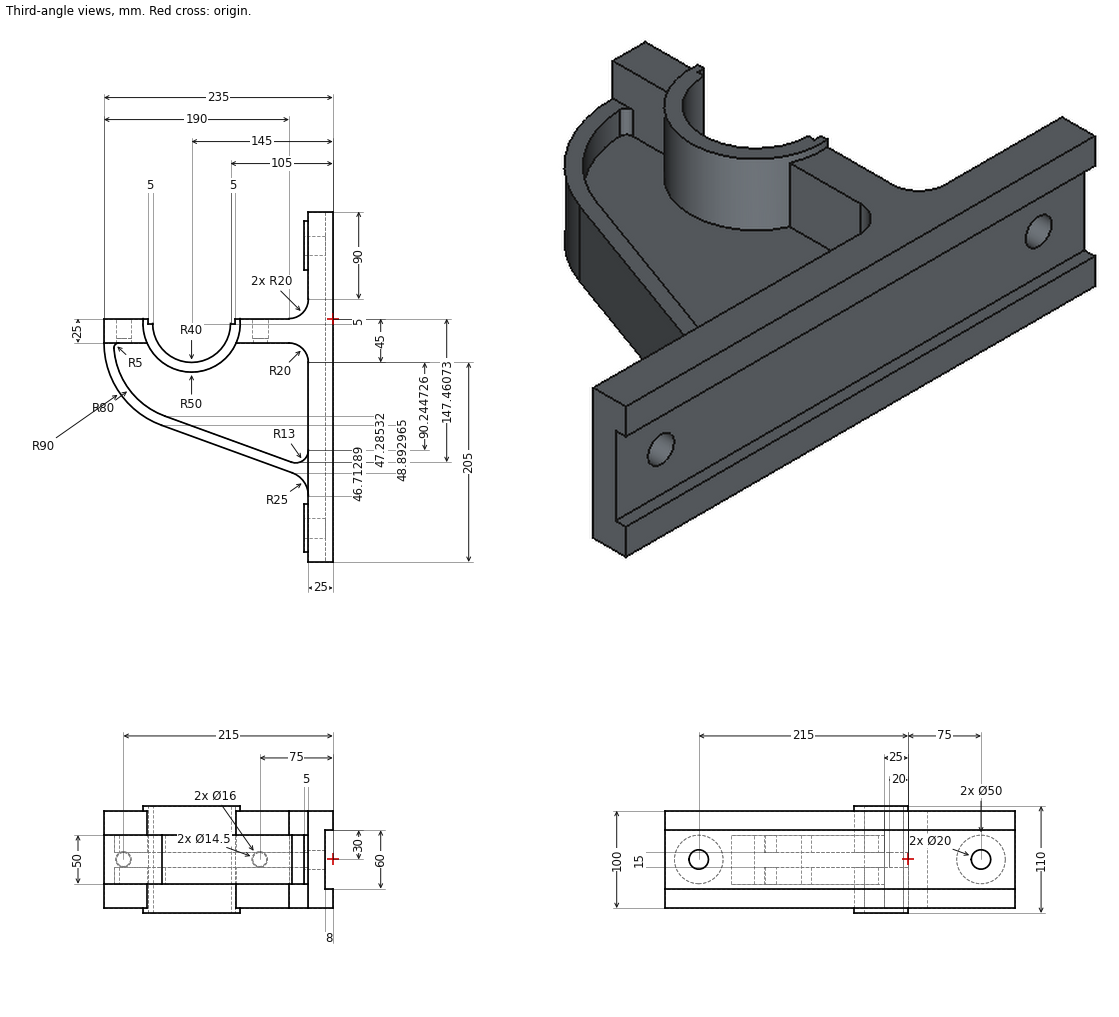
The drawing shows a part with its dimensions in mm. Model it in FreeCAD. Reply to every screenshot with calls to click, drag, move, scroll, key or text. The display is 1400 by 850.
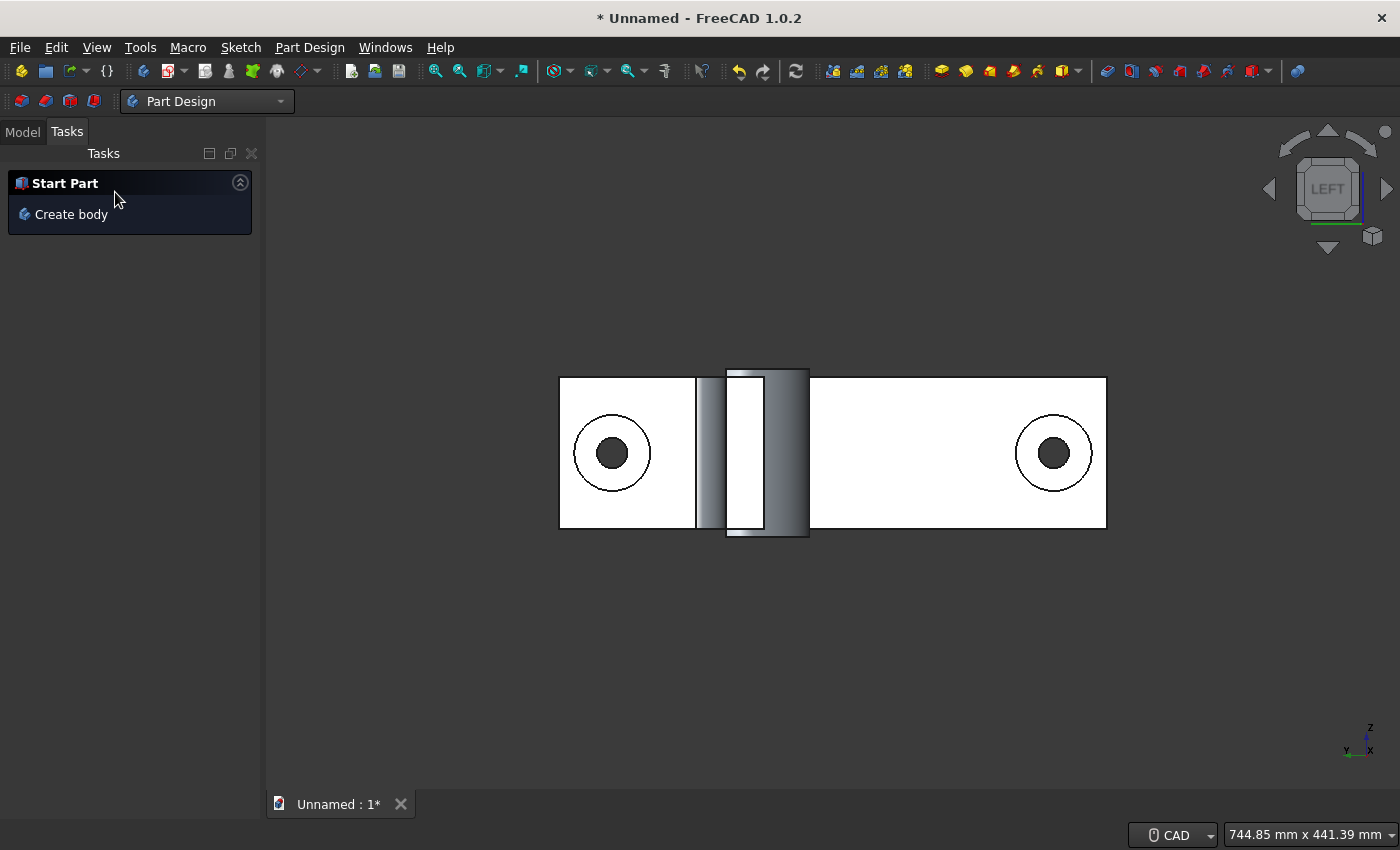
click(168, 72)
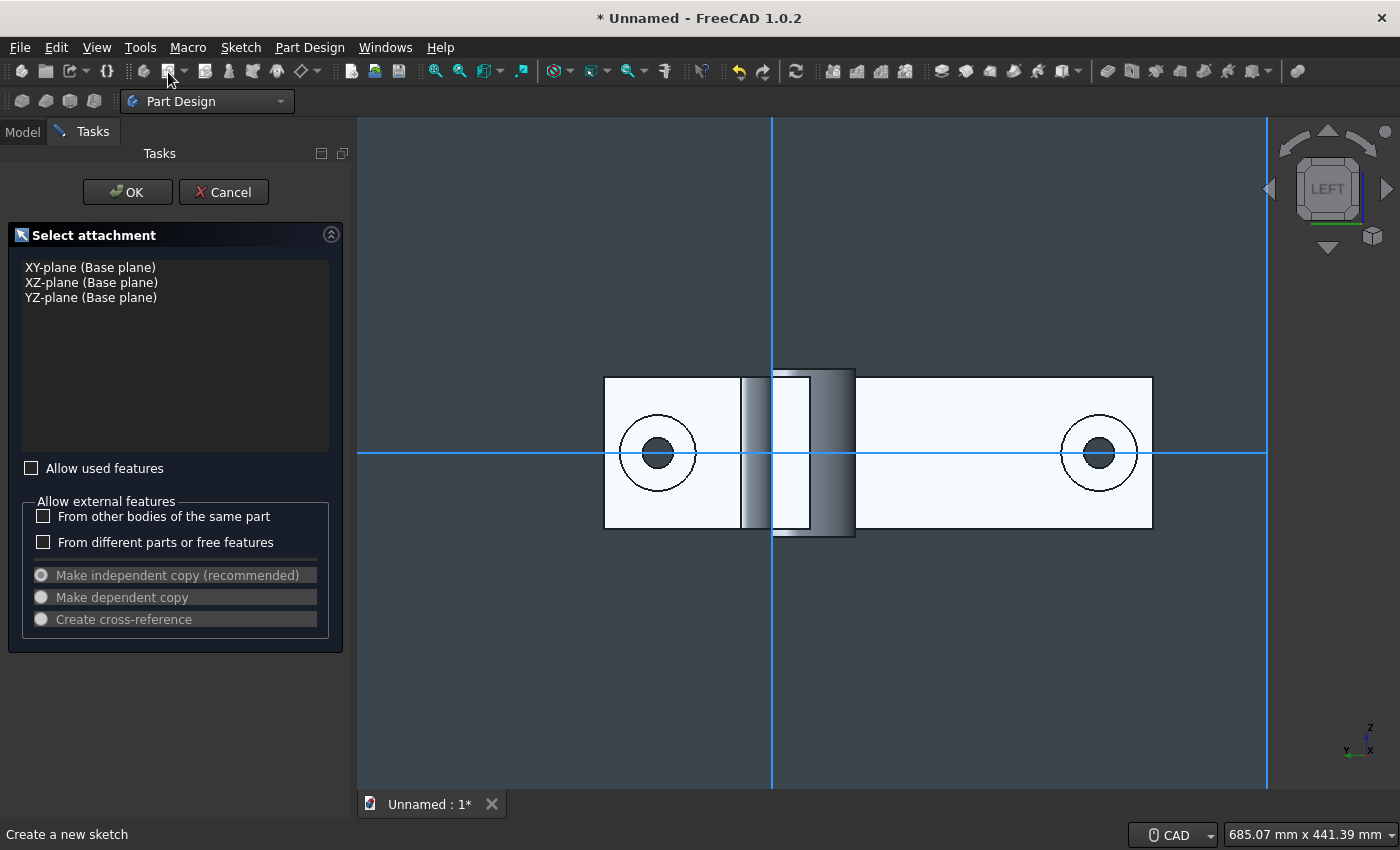
click(82, 268)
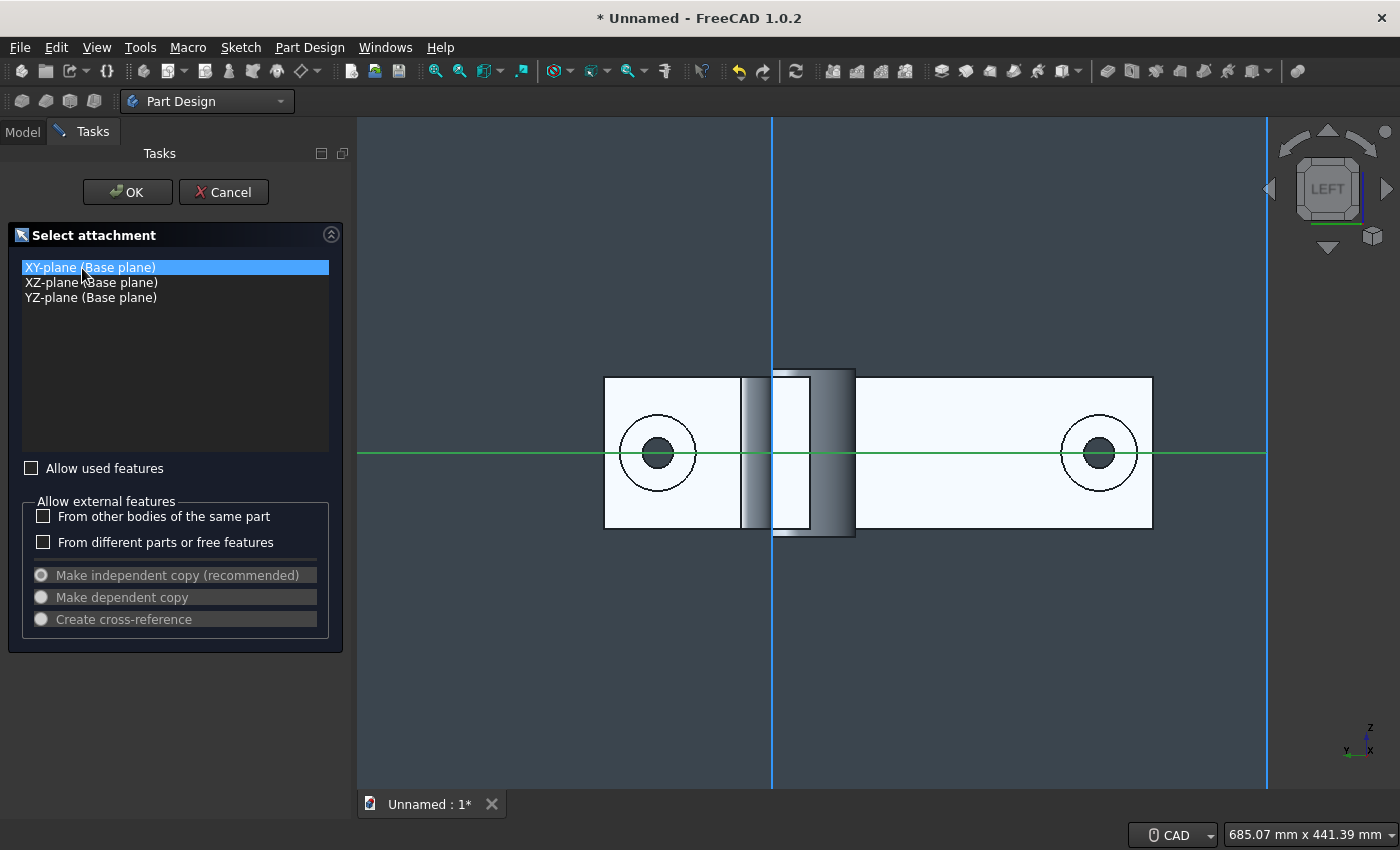
click(128, 192)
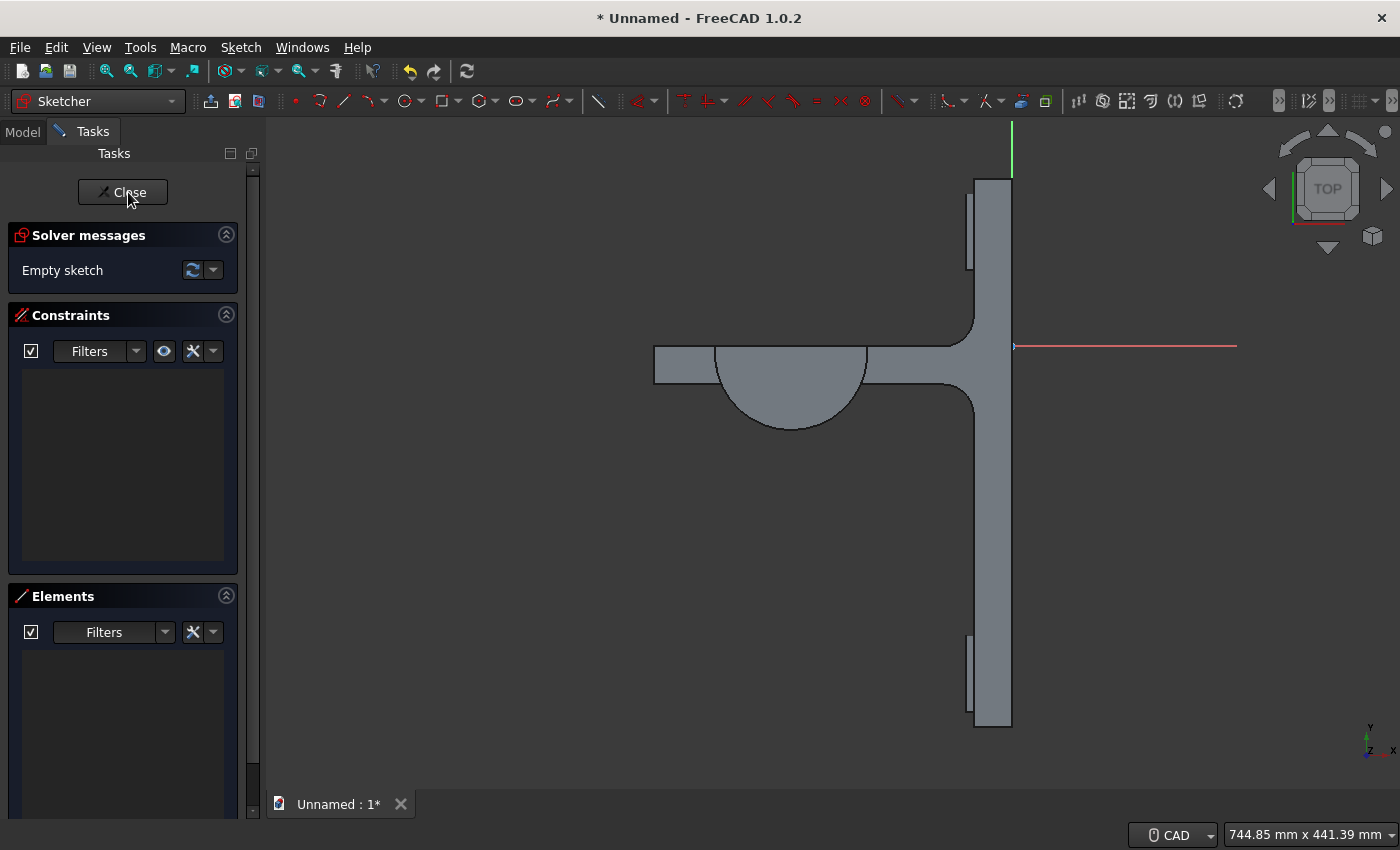
click(260, 102)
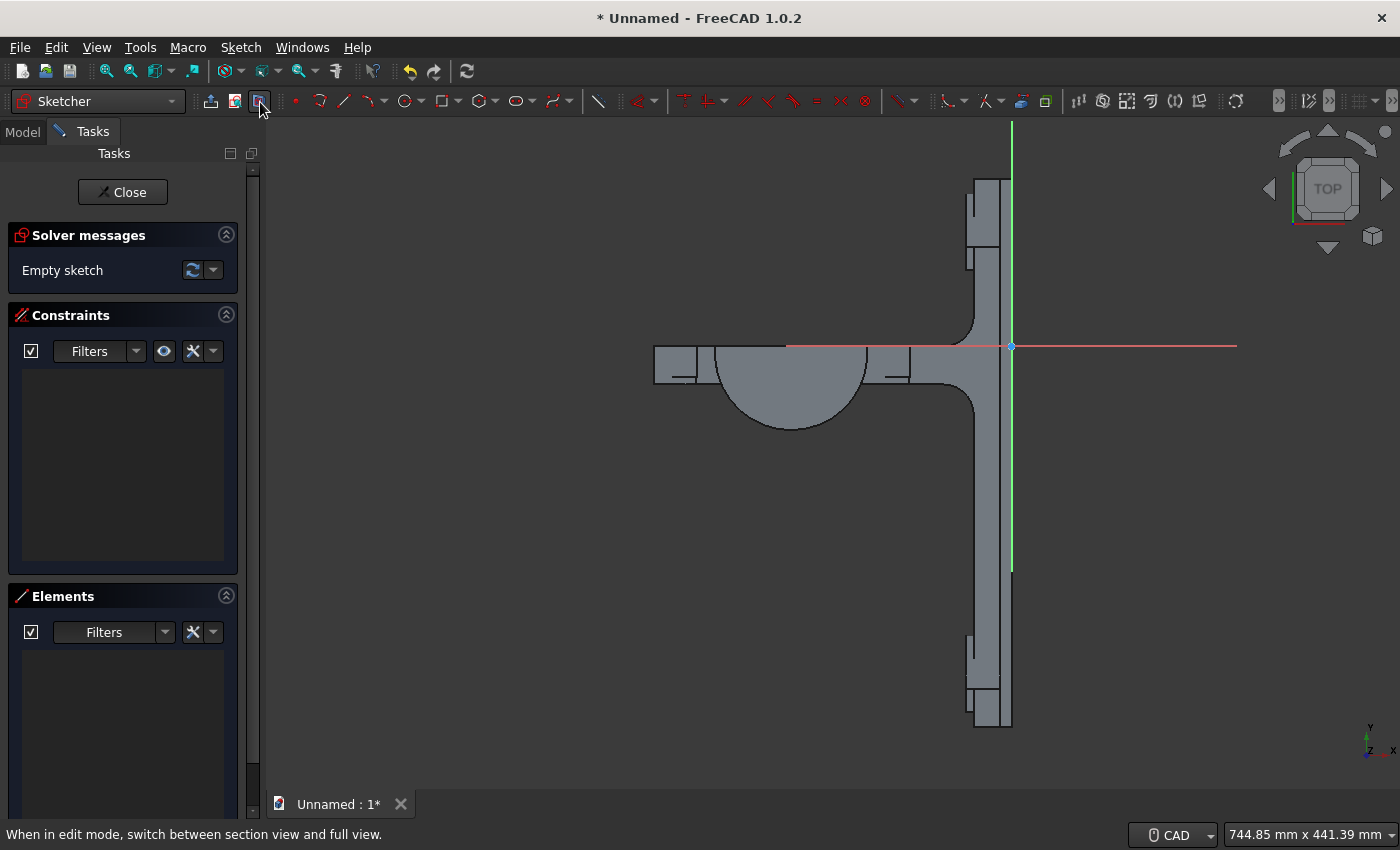
scroll(951, 322, up, 4)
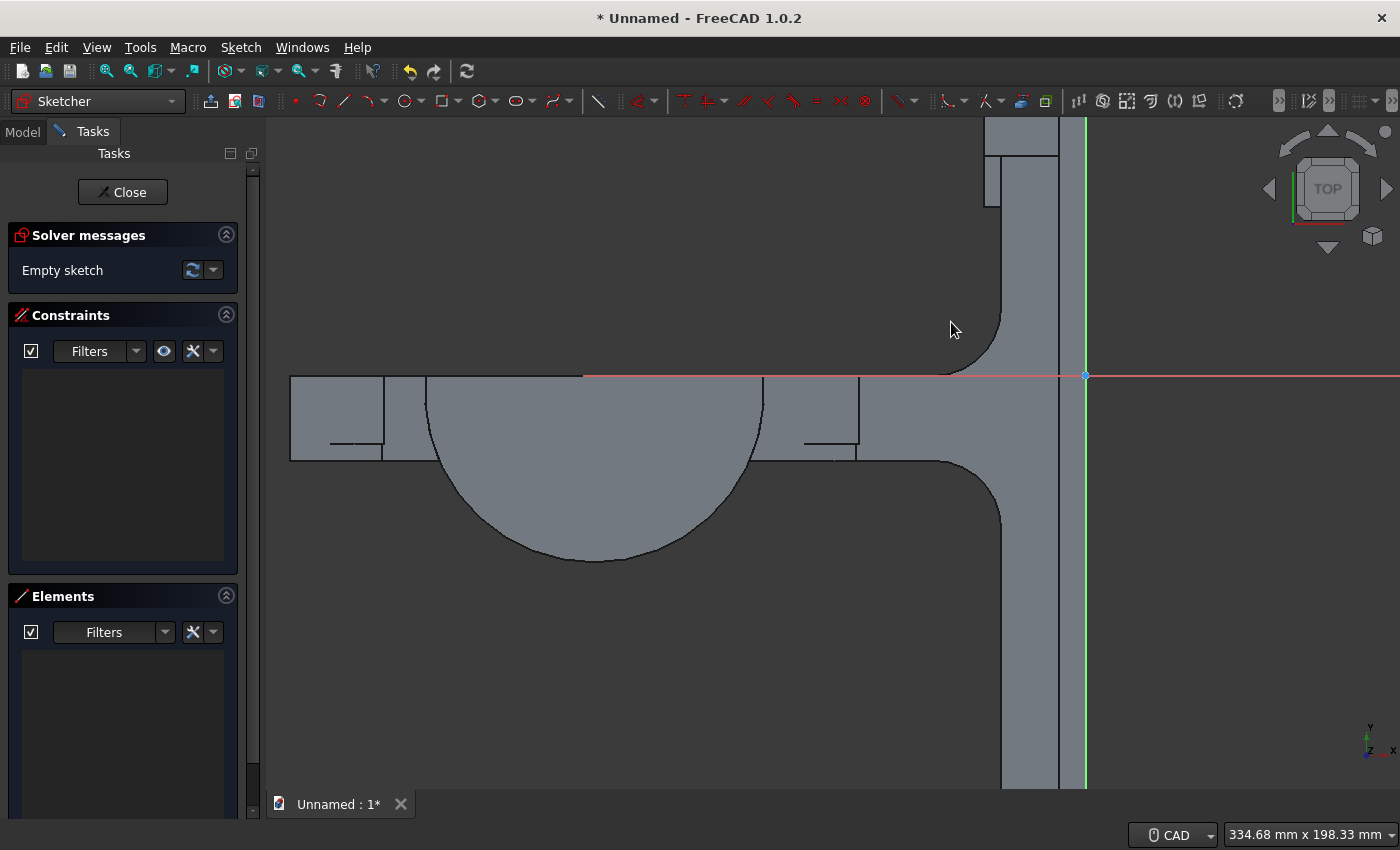
click(320, 102)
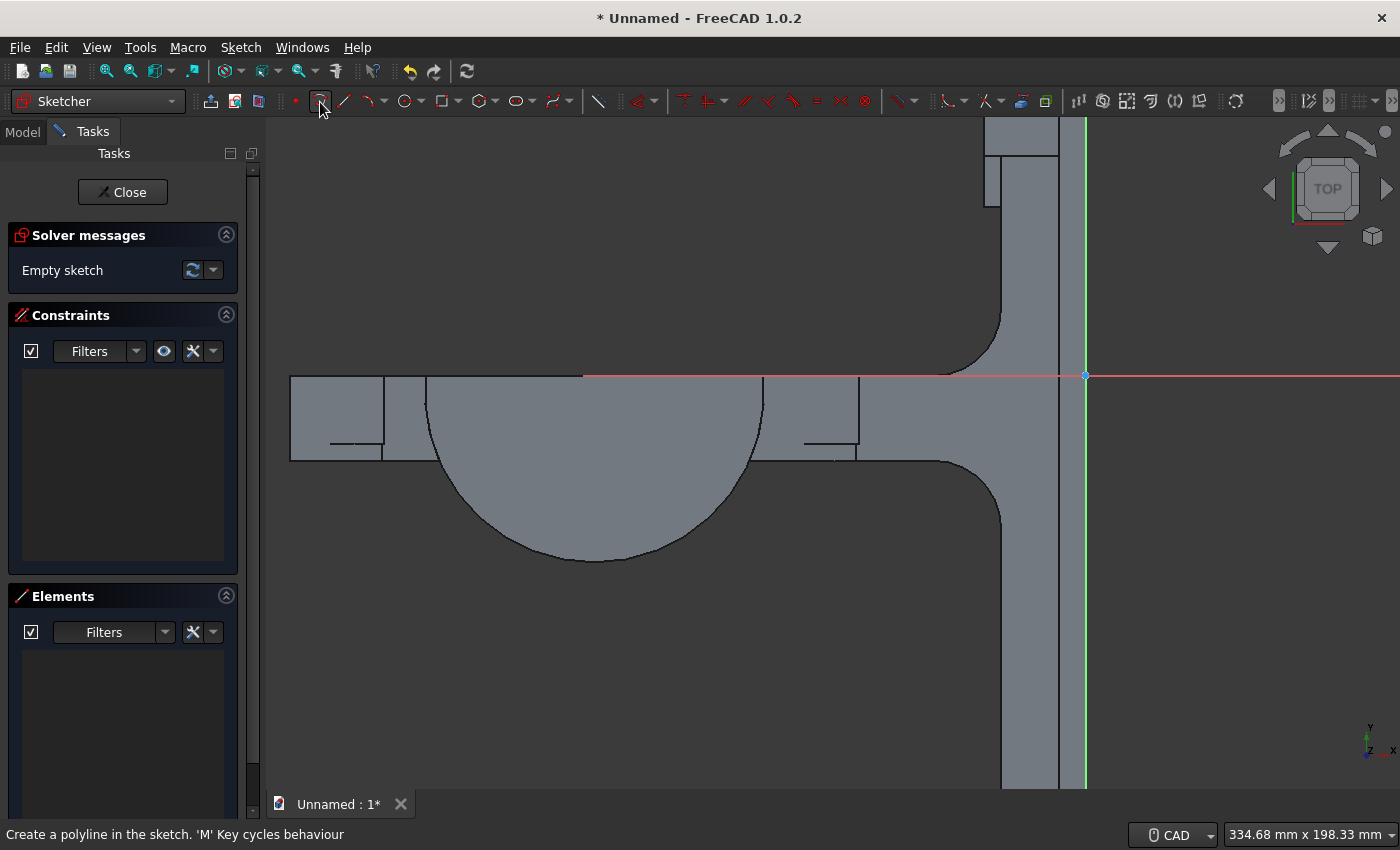
click(730, 393)
click(747, 393)
click(747, 376)
click(442, 385)
click(442, 393)
click(459, 393)
right_click(459, 393)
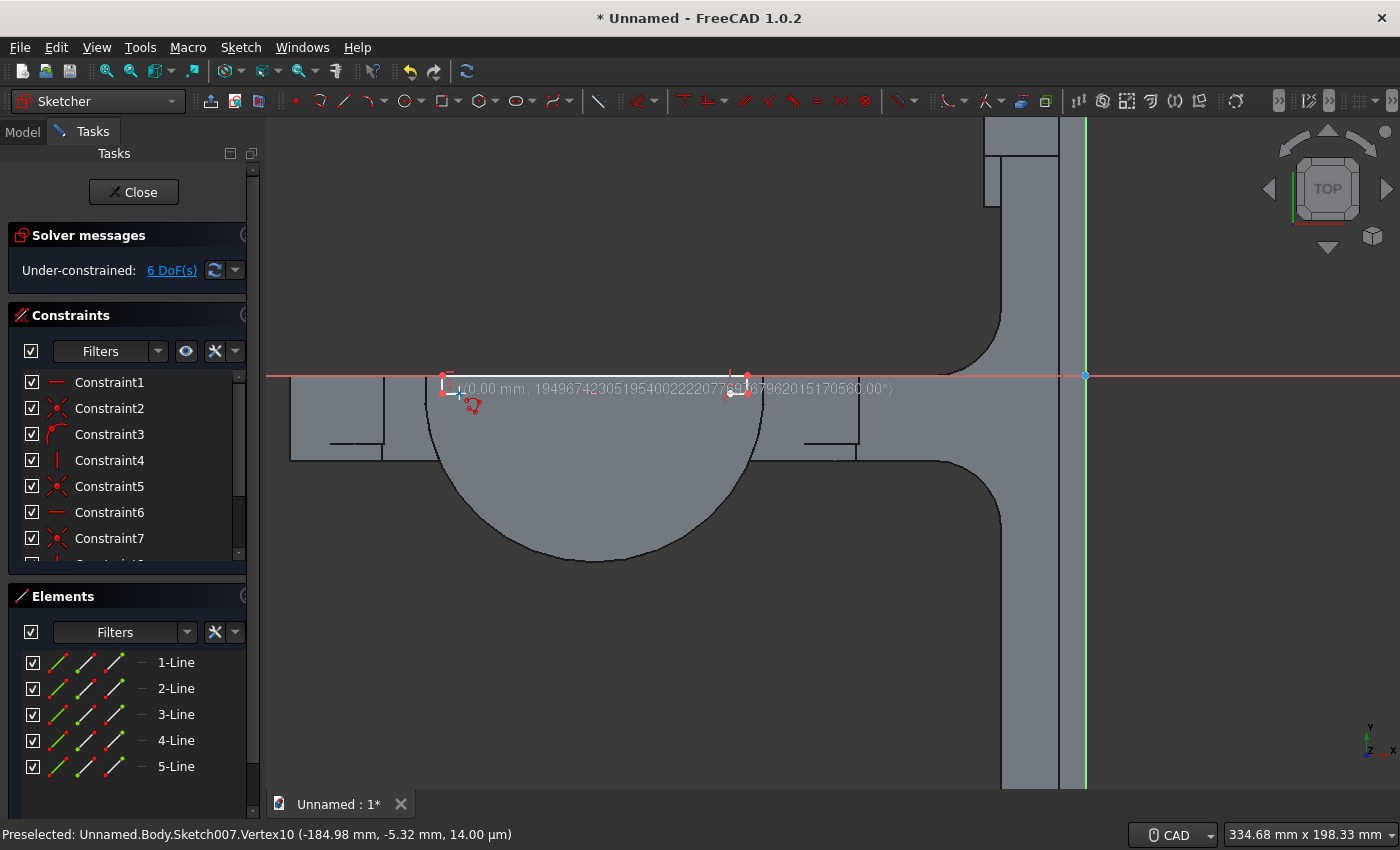
click(368, 102)